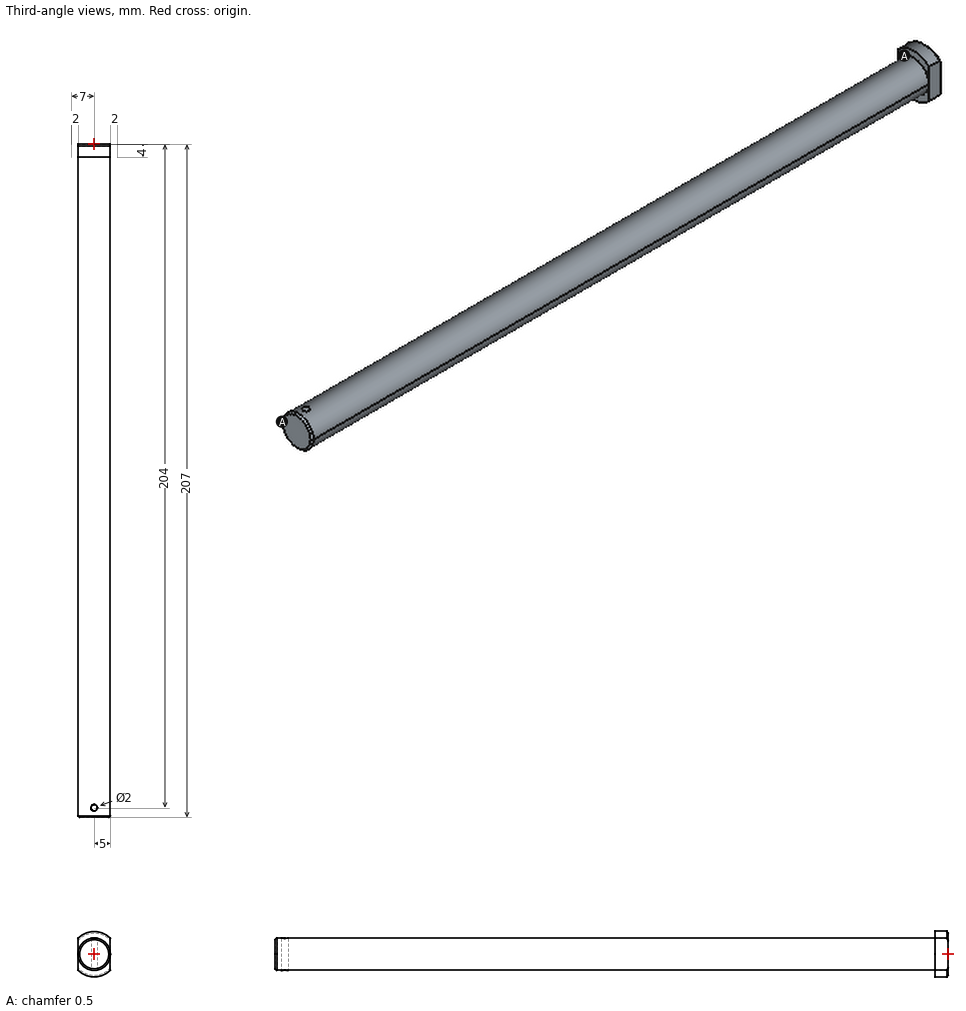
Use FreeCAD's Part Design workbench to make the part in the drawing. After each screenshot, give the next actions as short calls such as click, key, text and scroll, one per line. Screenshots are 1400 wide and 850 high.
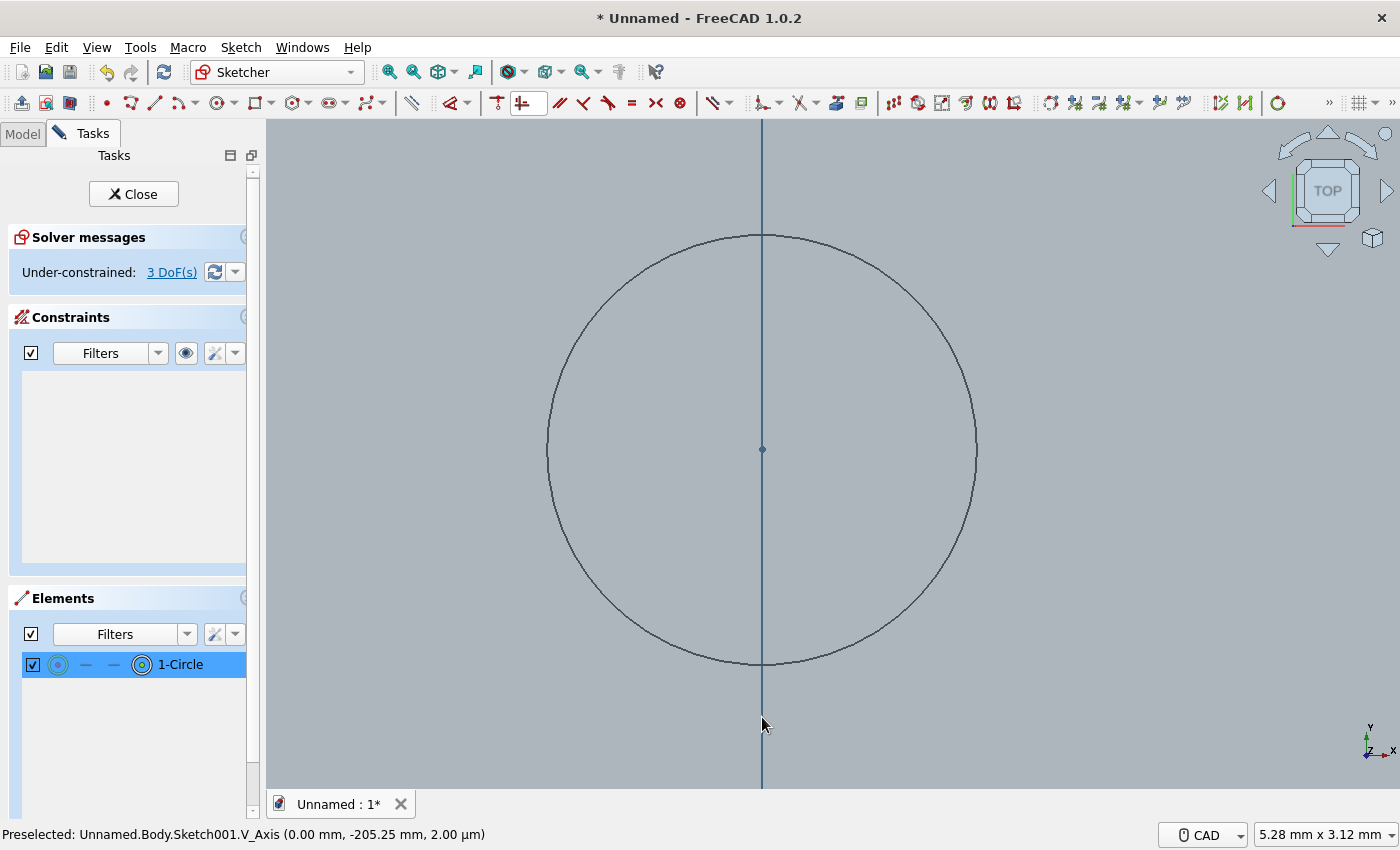
click(498, 104)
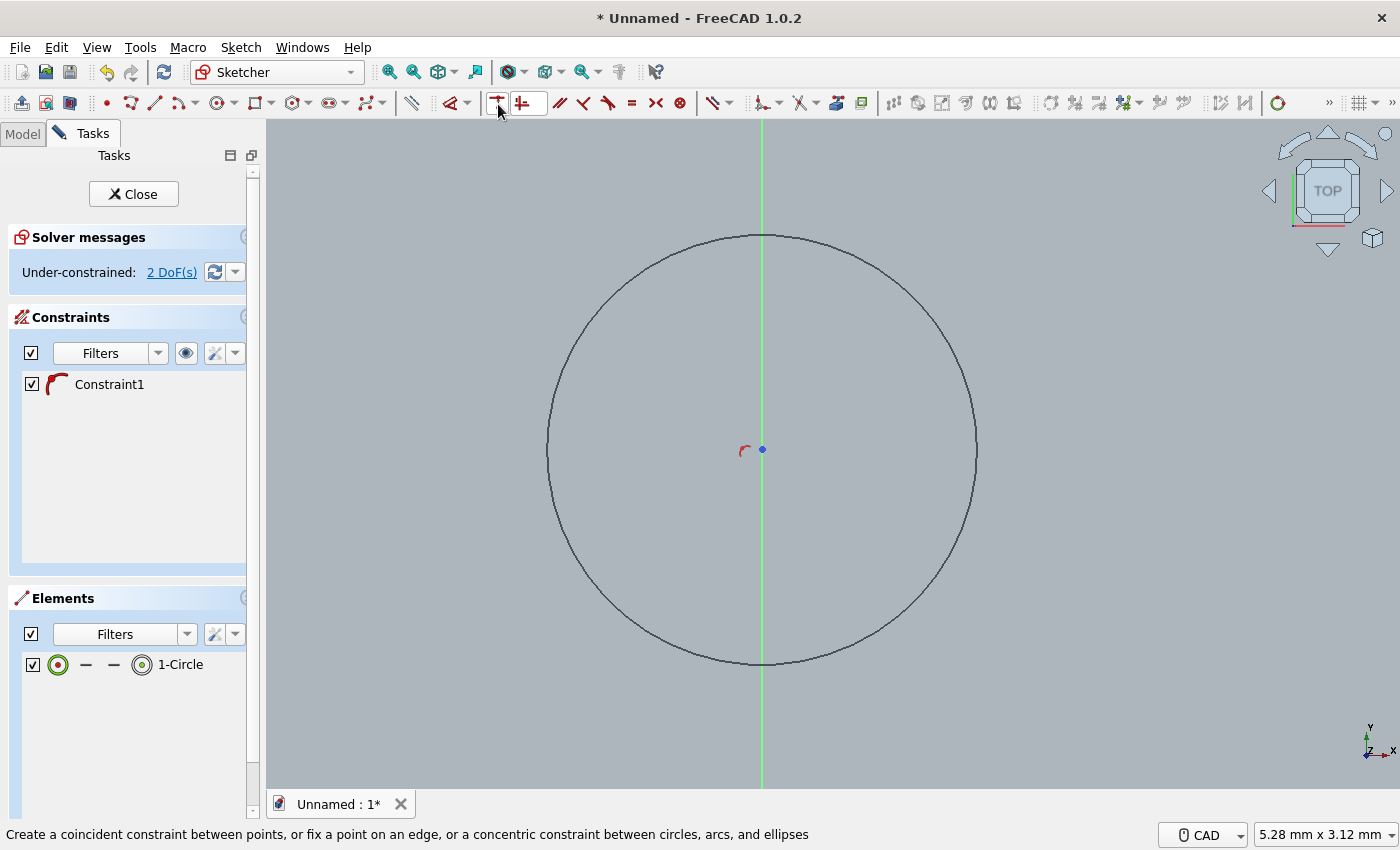
click(450, 104)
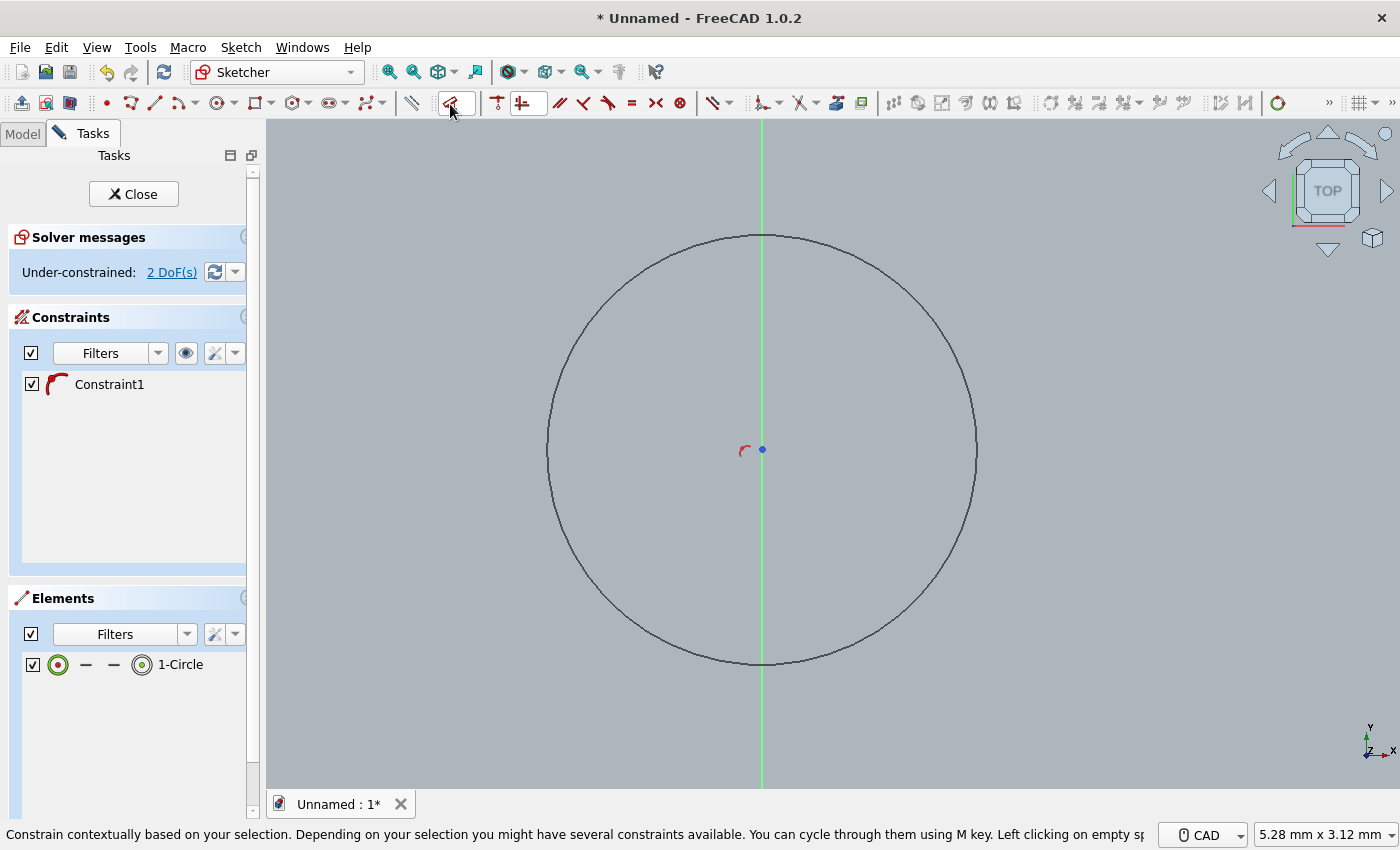
click(914, 298)
click(937, 275)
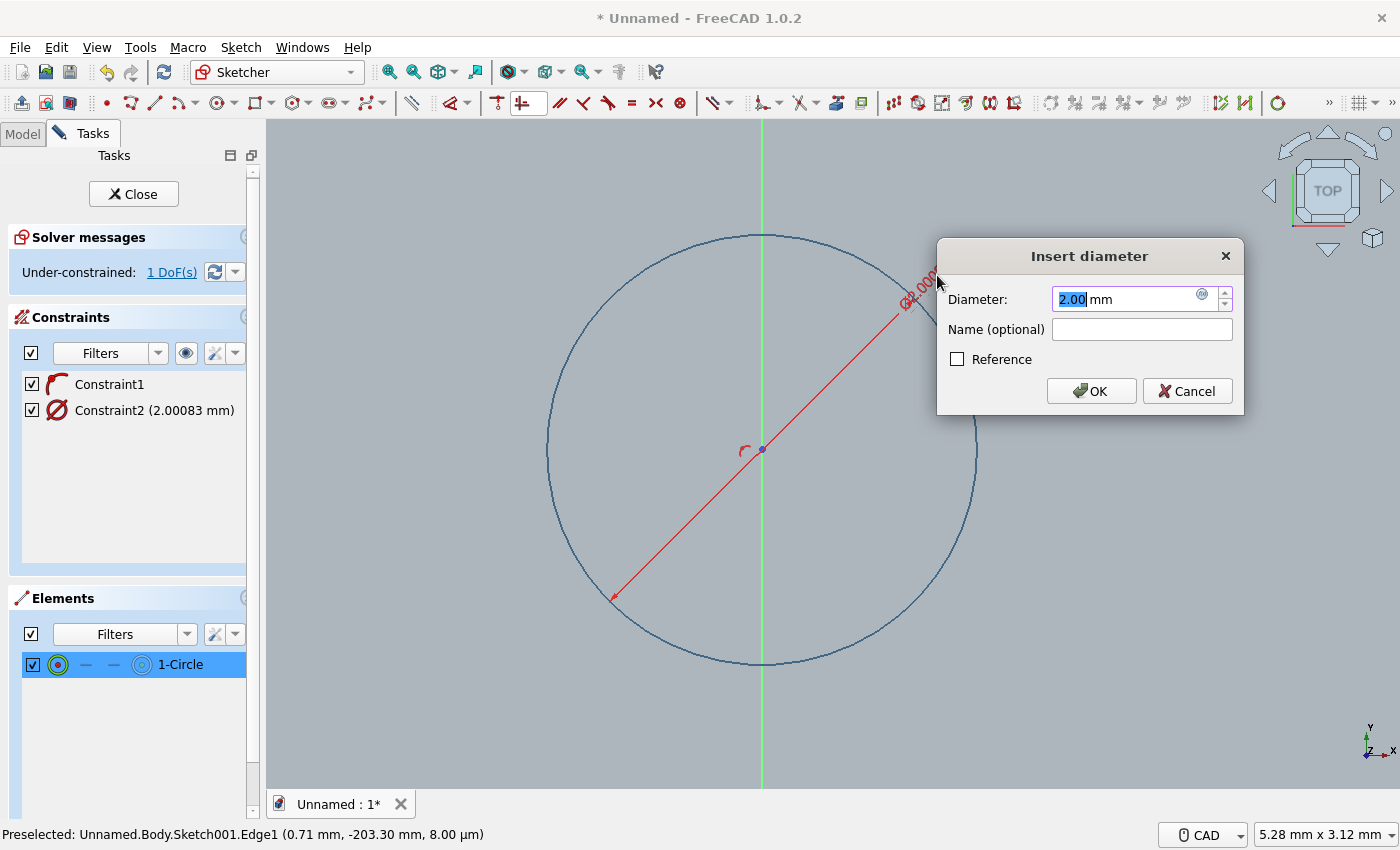
text(2)
key(Return)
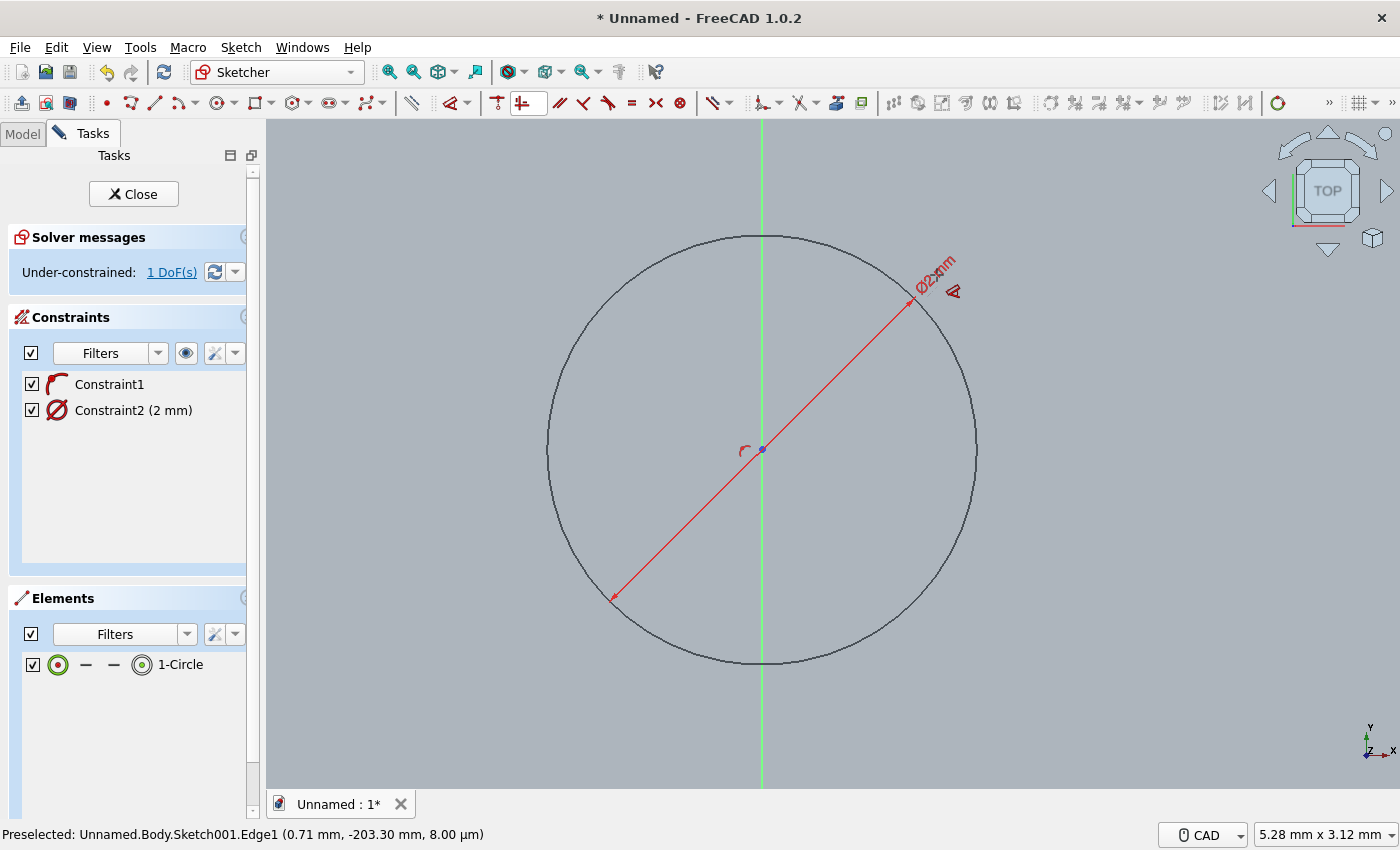
click(762, 450)
click(796, 299)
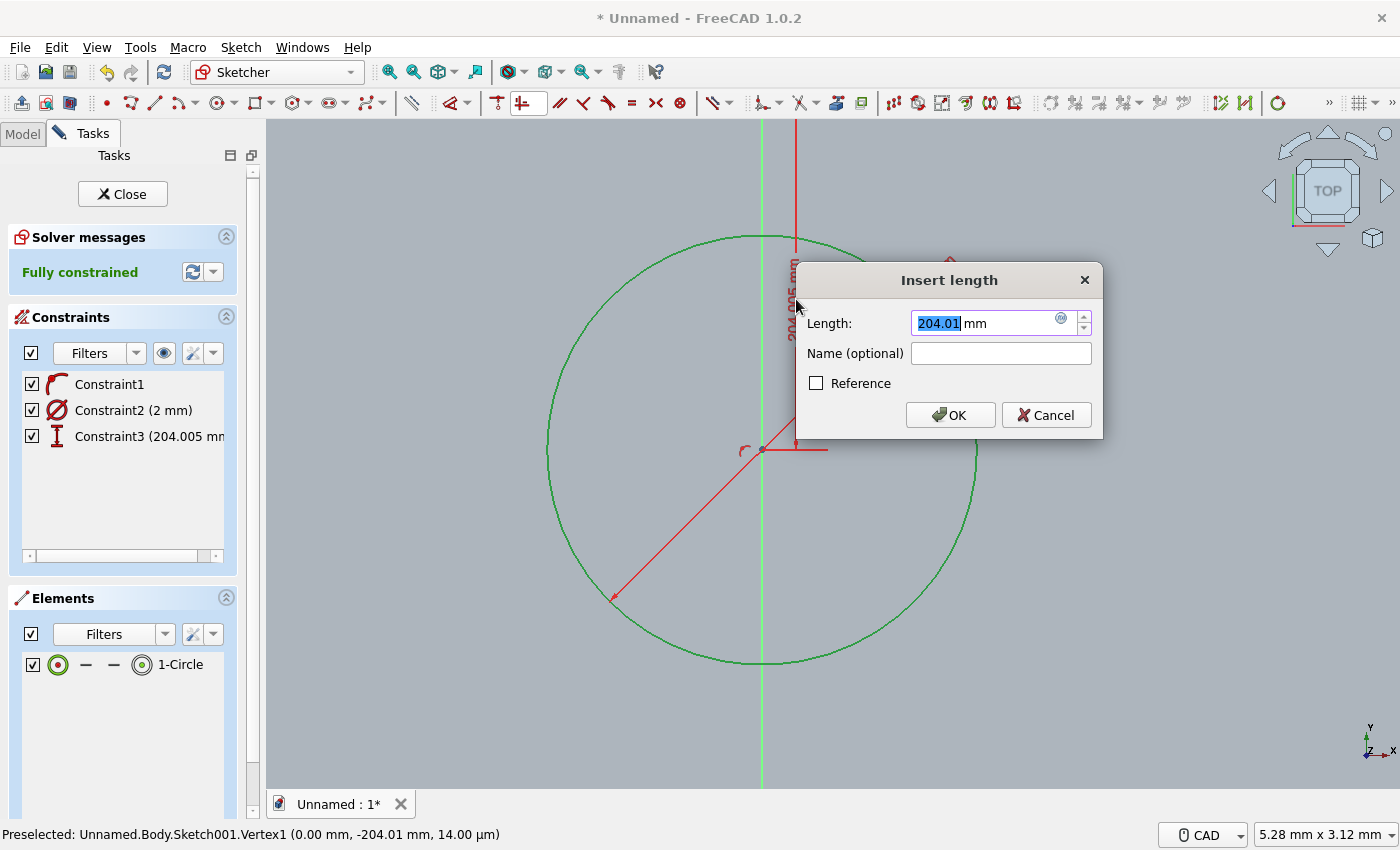
text(204)
key(Return)
key(Escape)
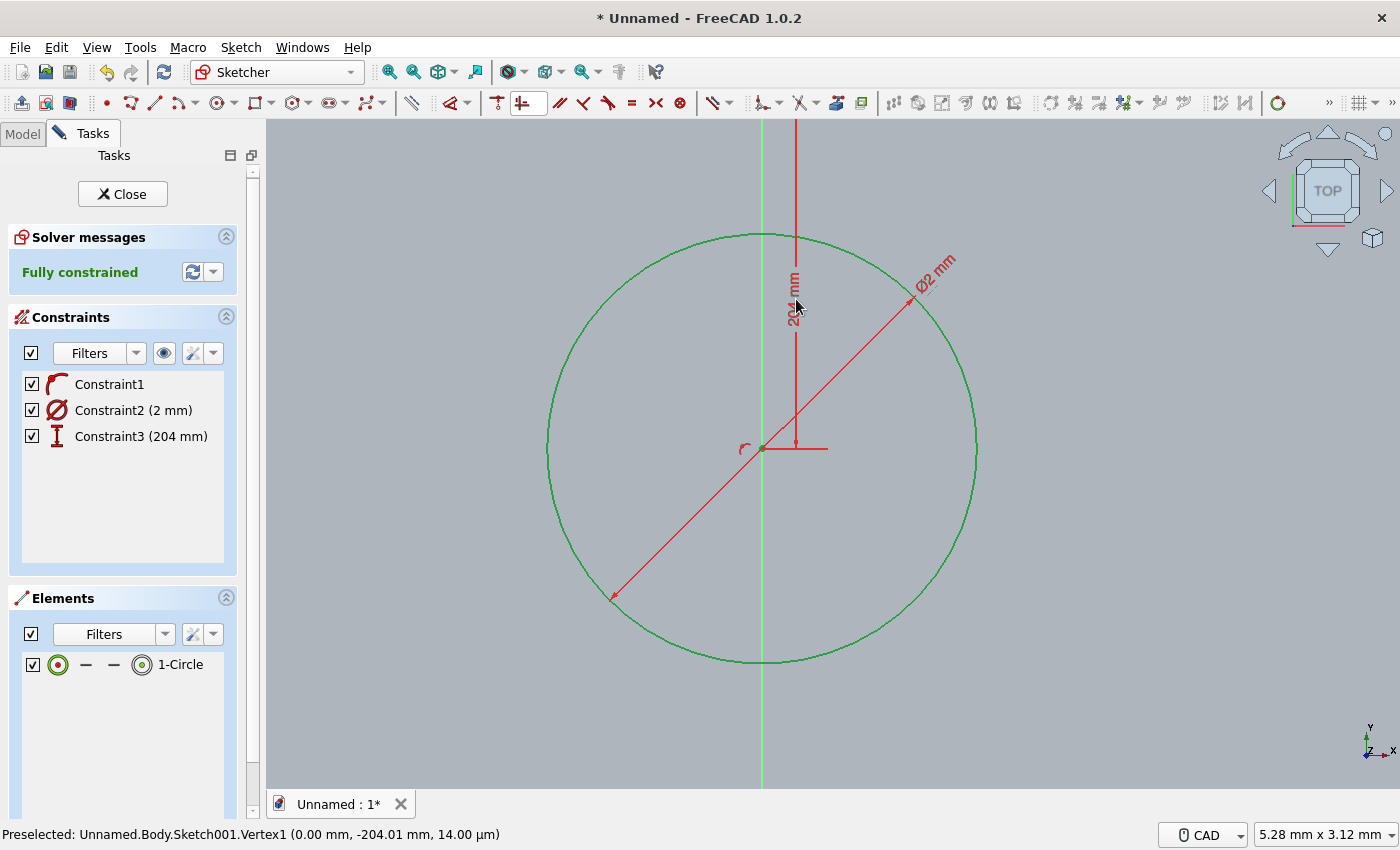
click(123, 194)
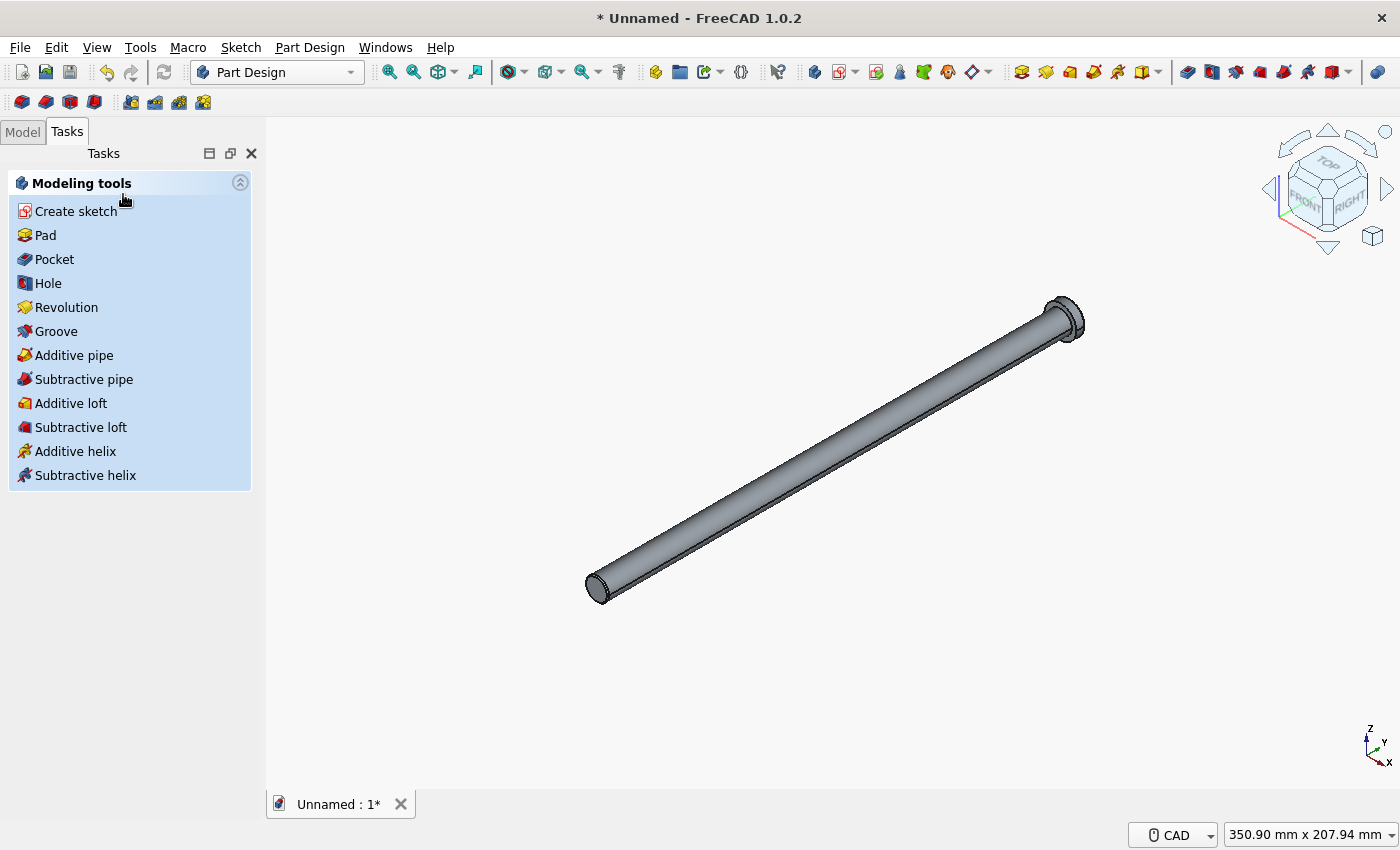
click(1188, 72)